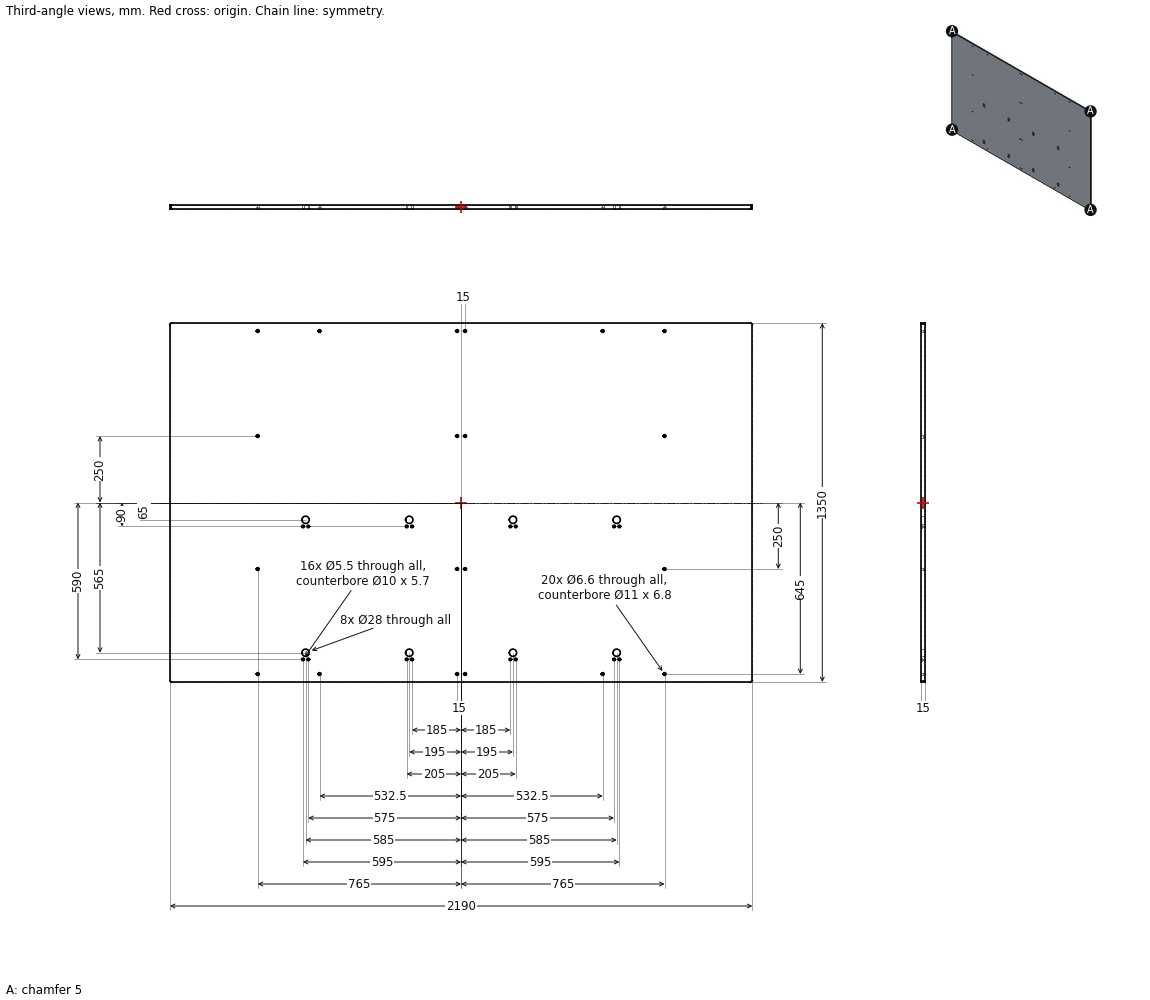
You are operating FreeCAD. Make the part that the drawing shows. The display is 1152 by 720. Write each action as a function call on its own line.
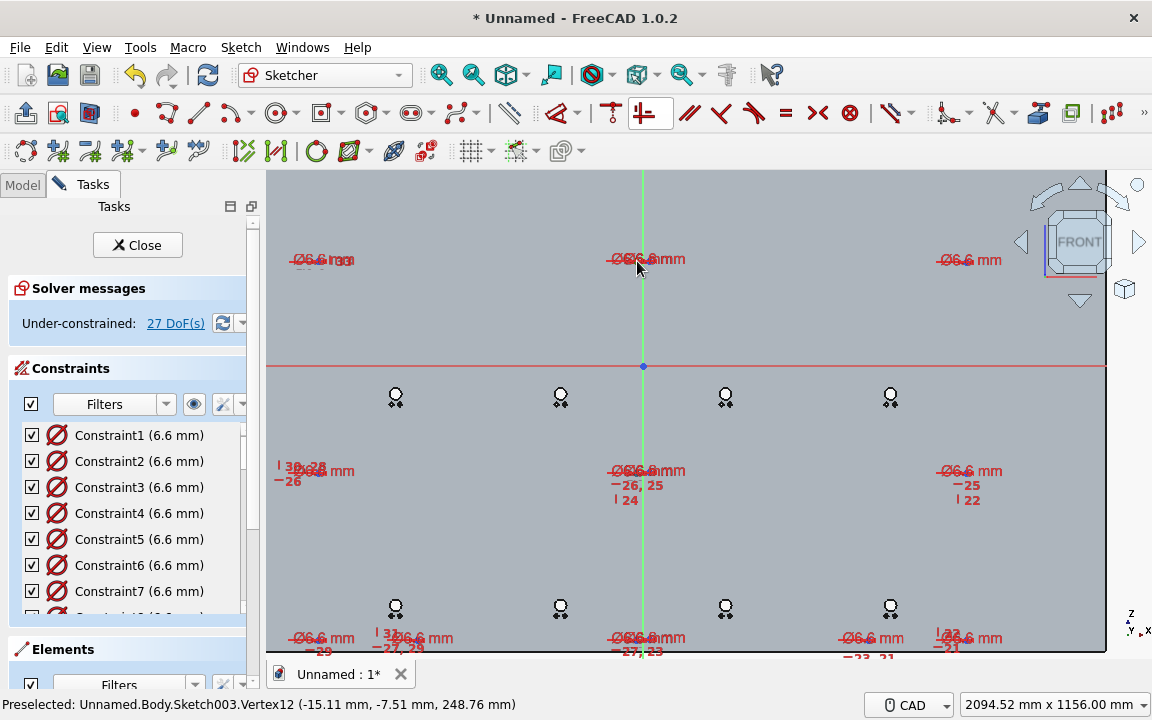
key(v)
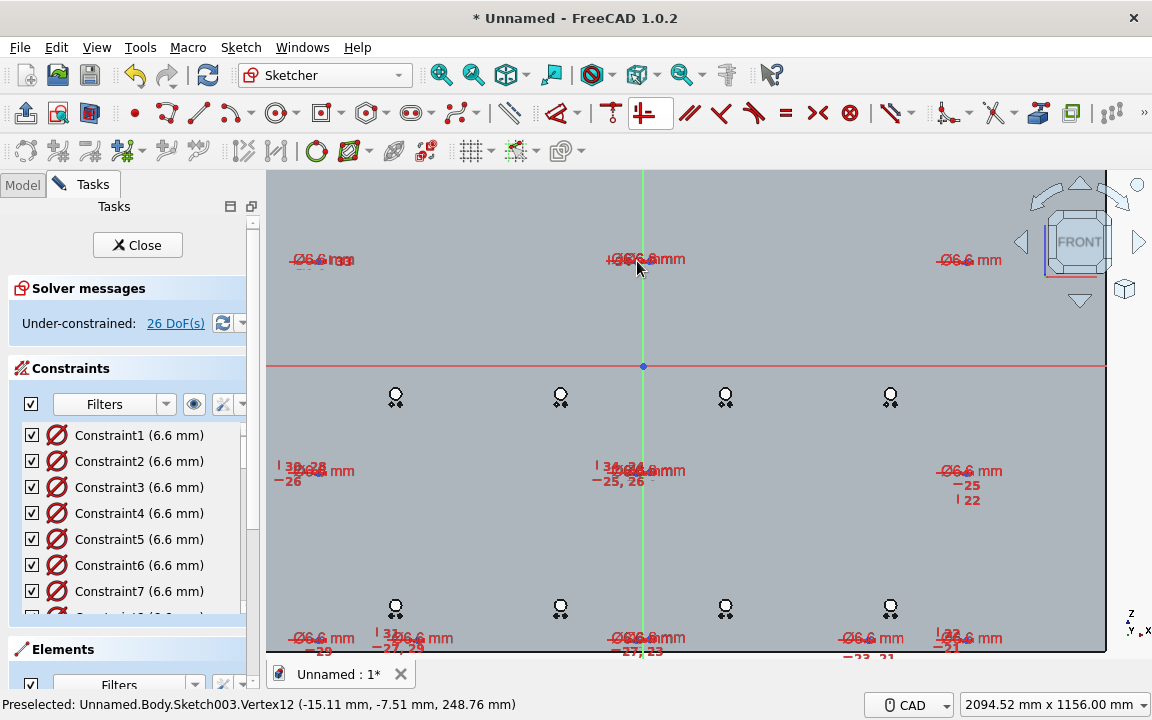
click(319, 262)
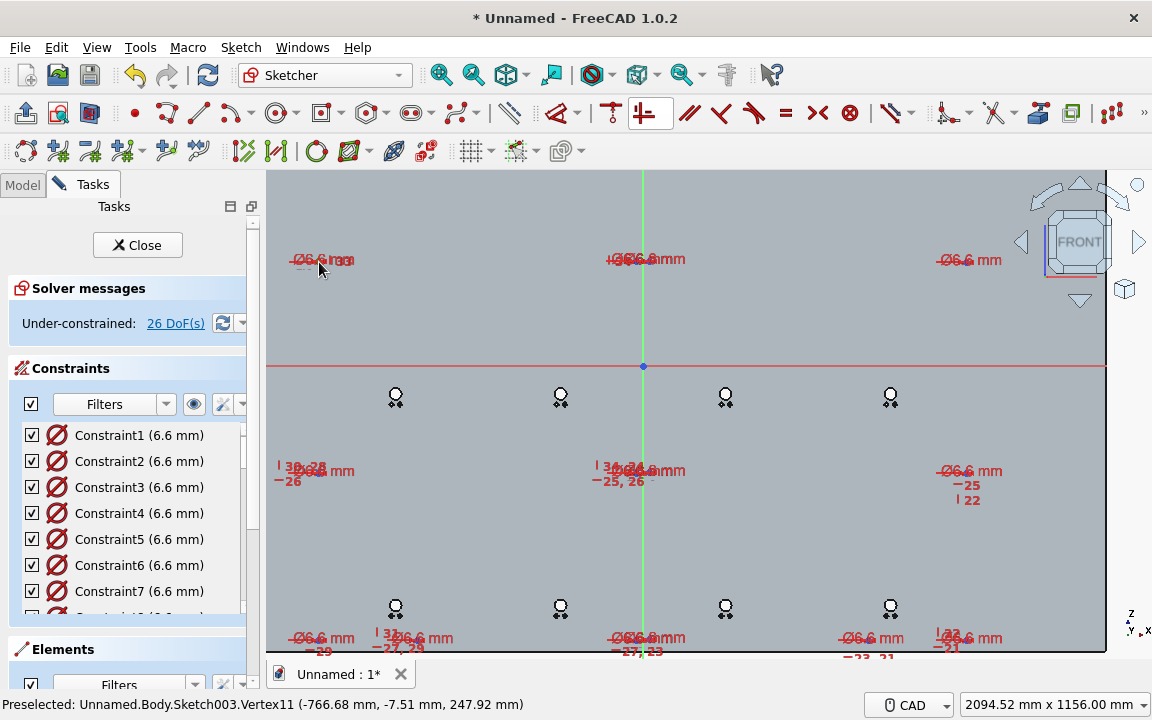
click(637, 261)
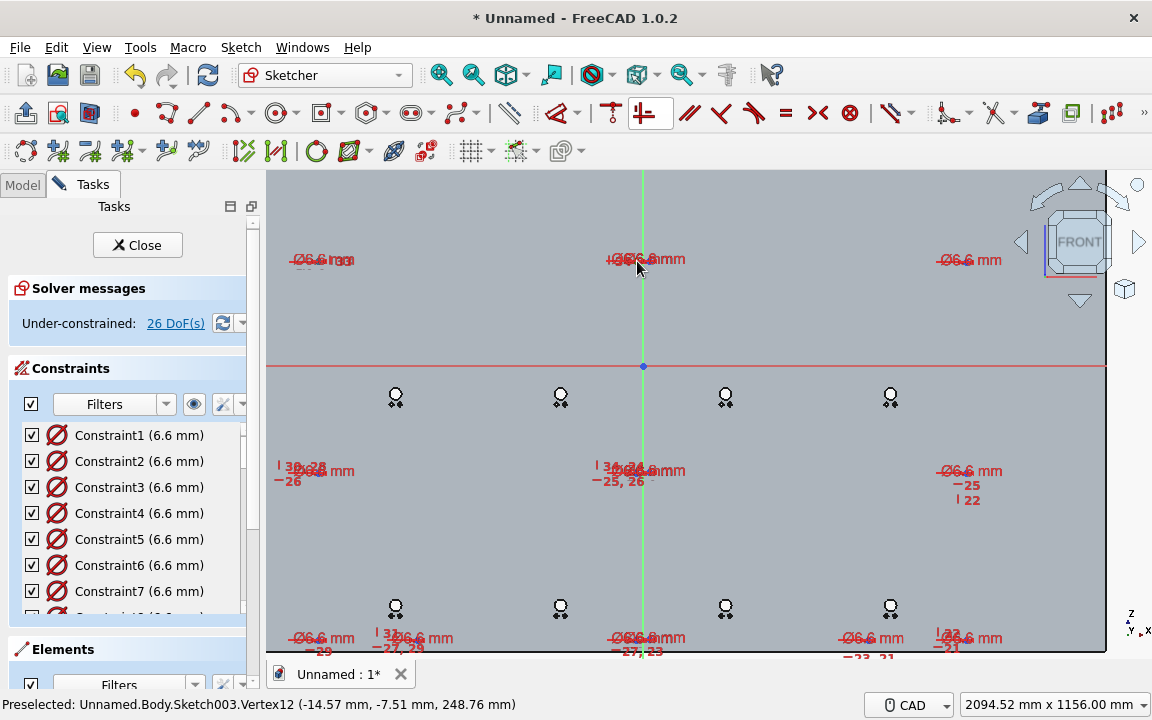
key(h)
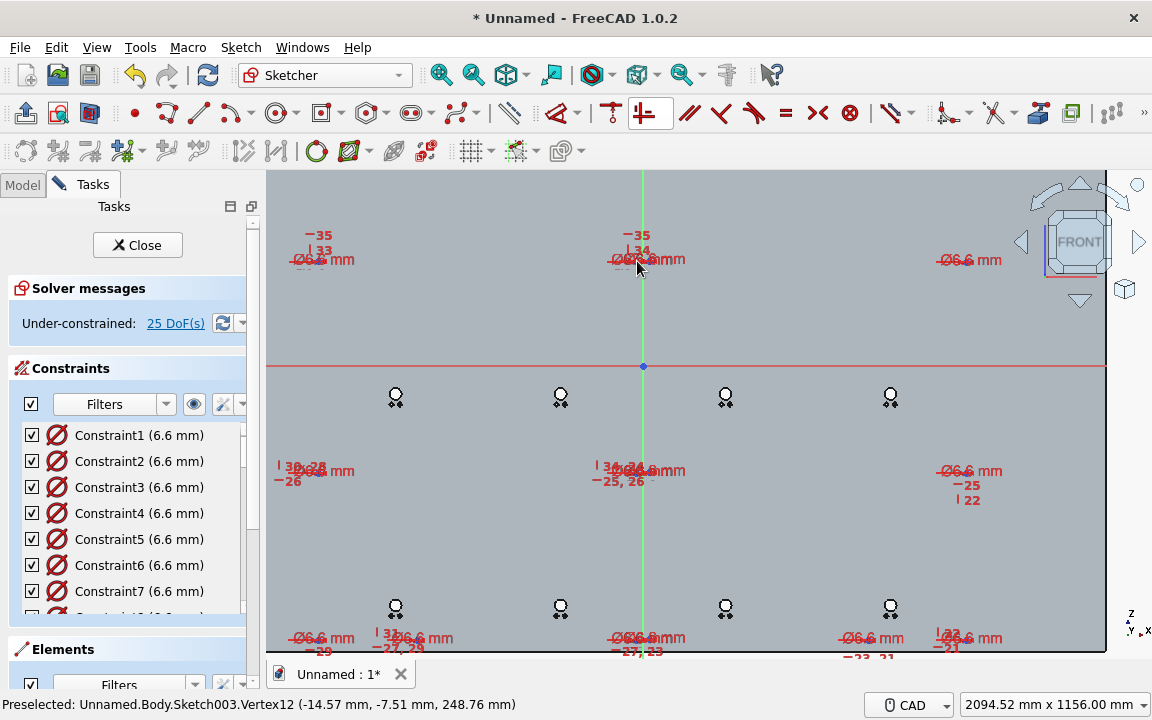
click(637, 262)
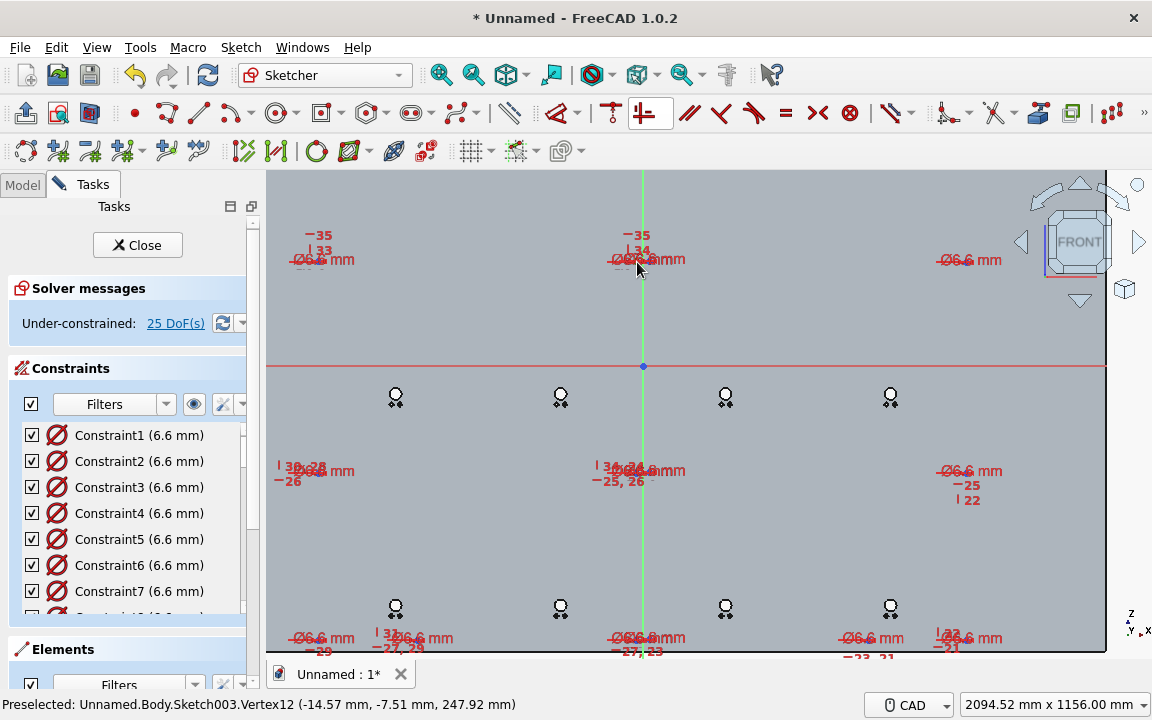
scroll(637, 473, down, 3)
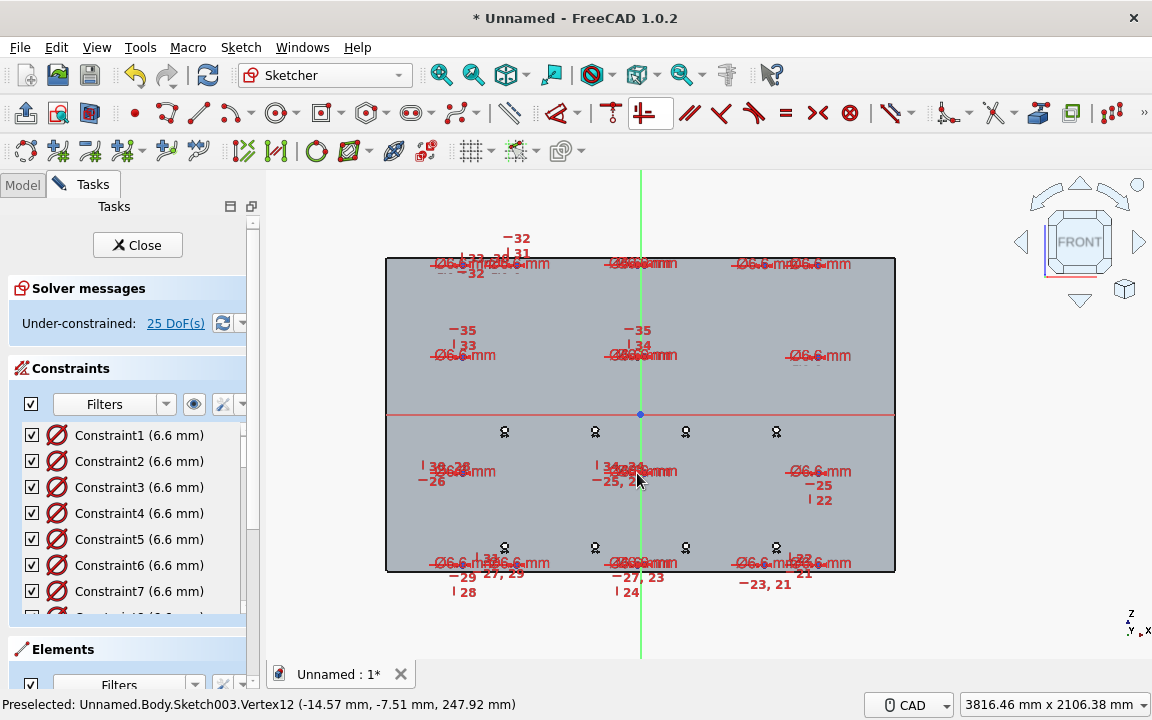
scroll(637, 265, up, 3)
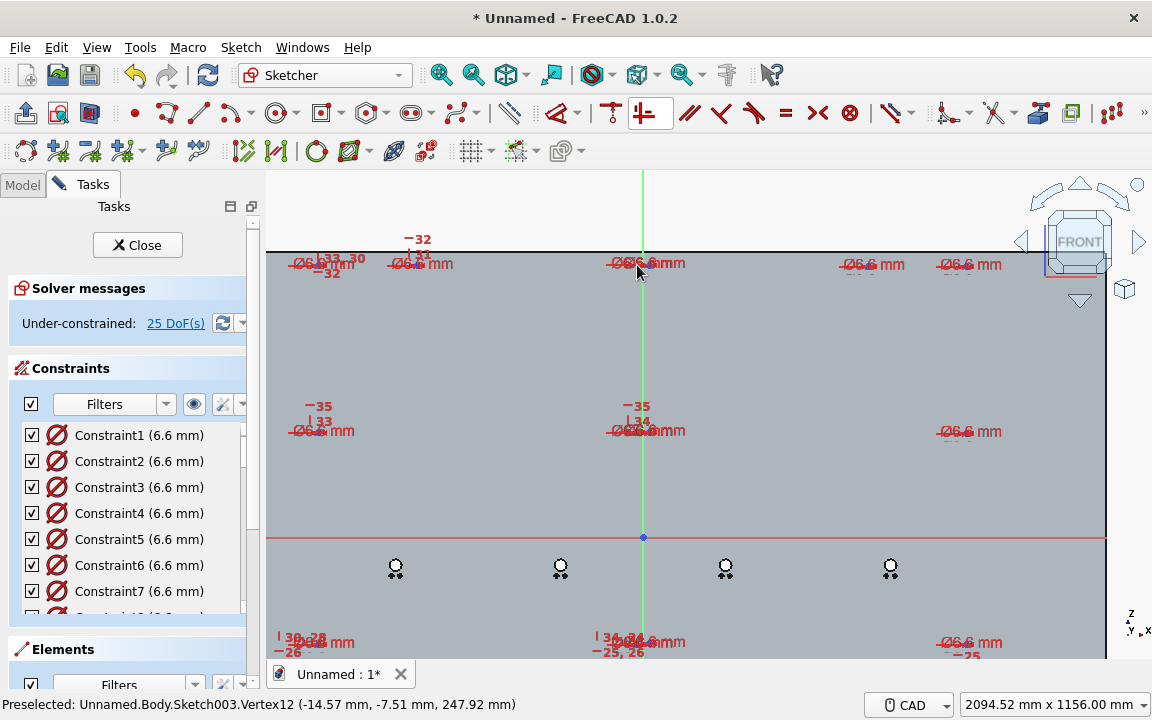
click(637, 265)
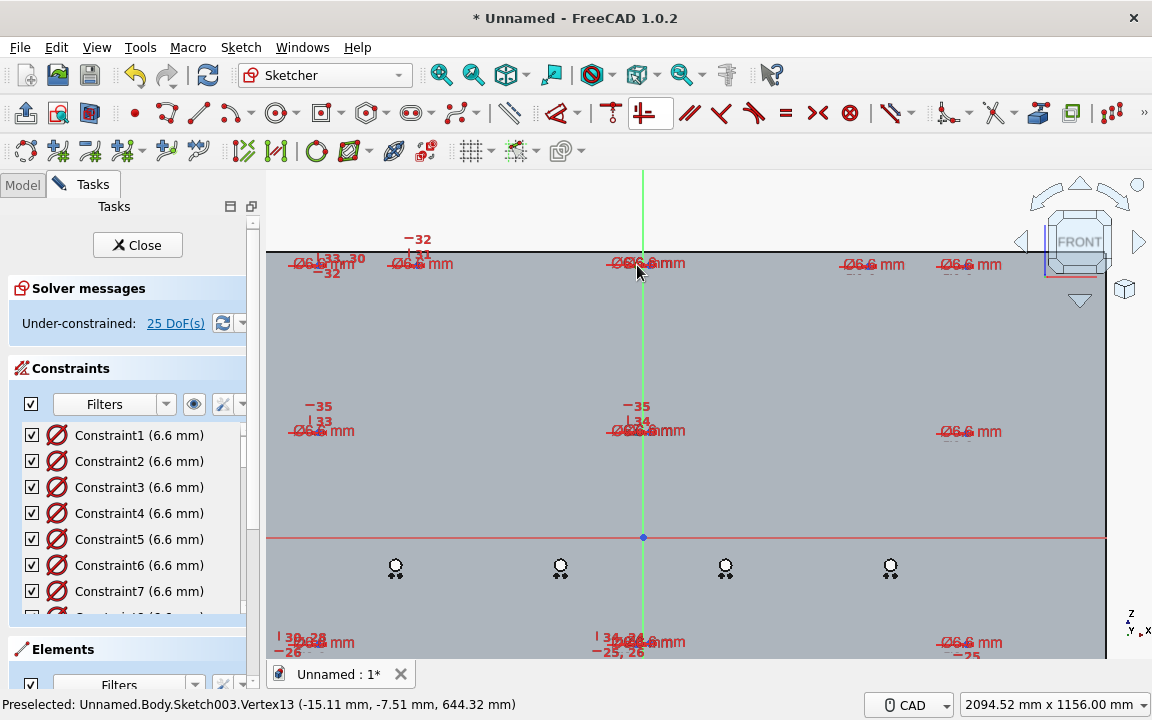
key(v)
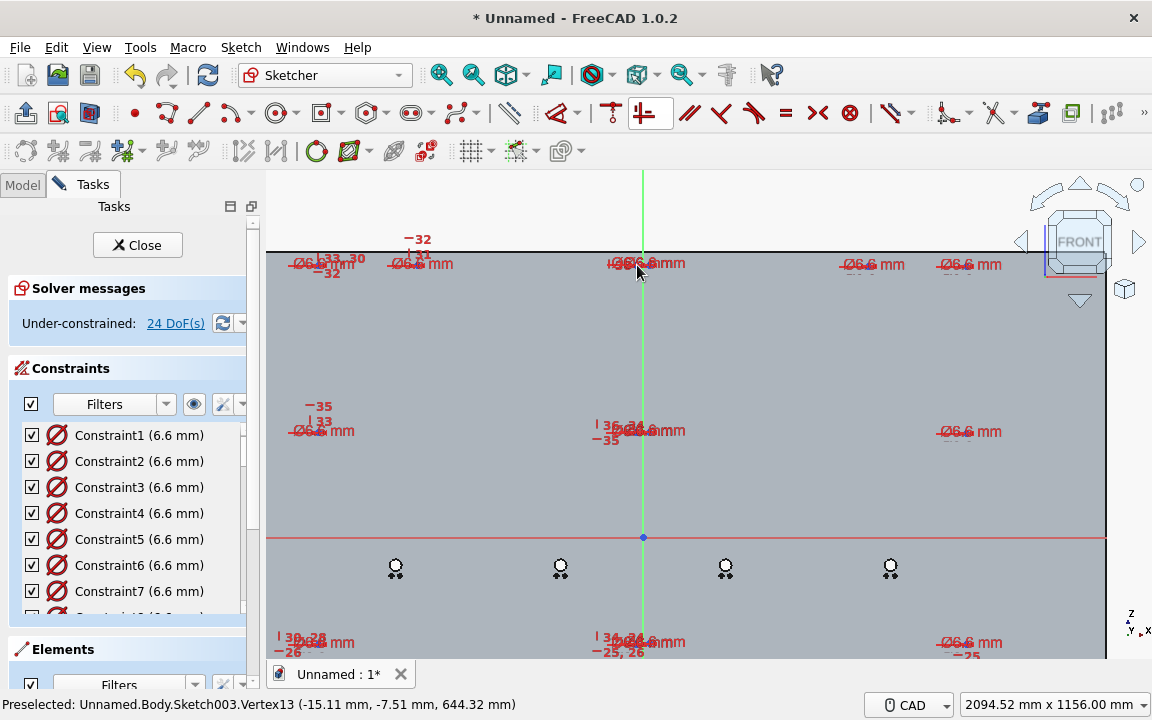
click(417, 266)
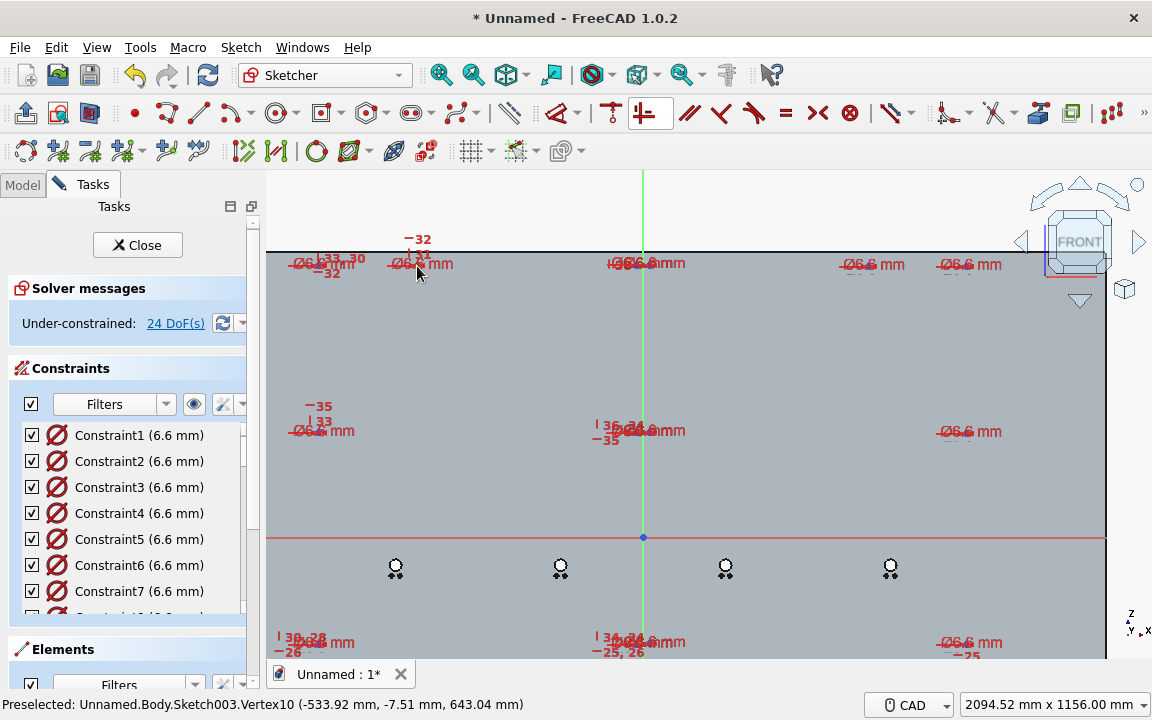
click(637, 265)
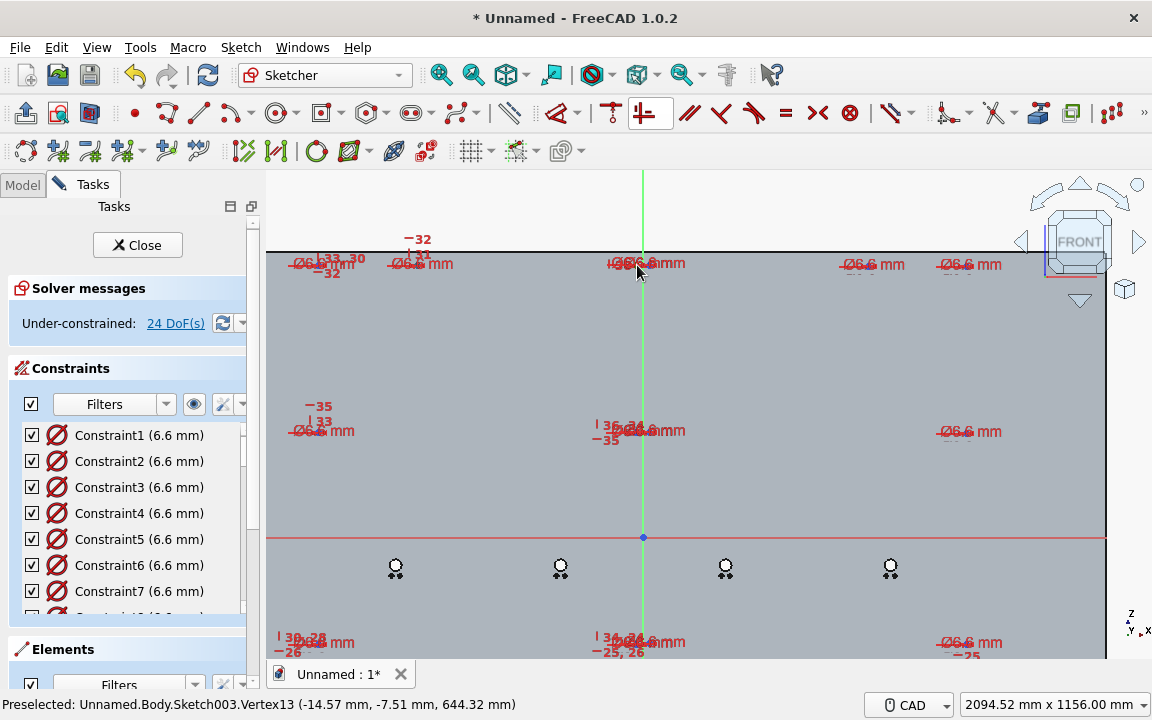
key(h)